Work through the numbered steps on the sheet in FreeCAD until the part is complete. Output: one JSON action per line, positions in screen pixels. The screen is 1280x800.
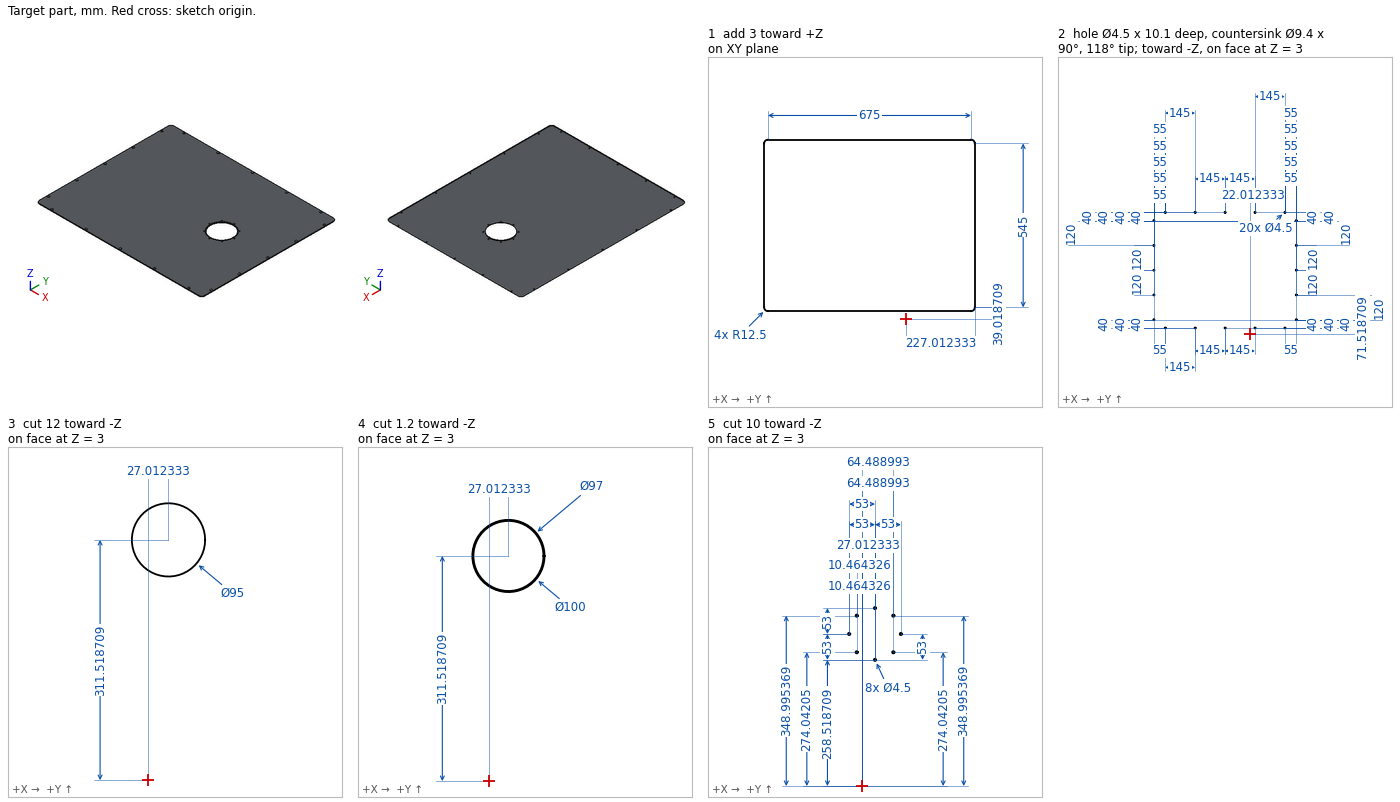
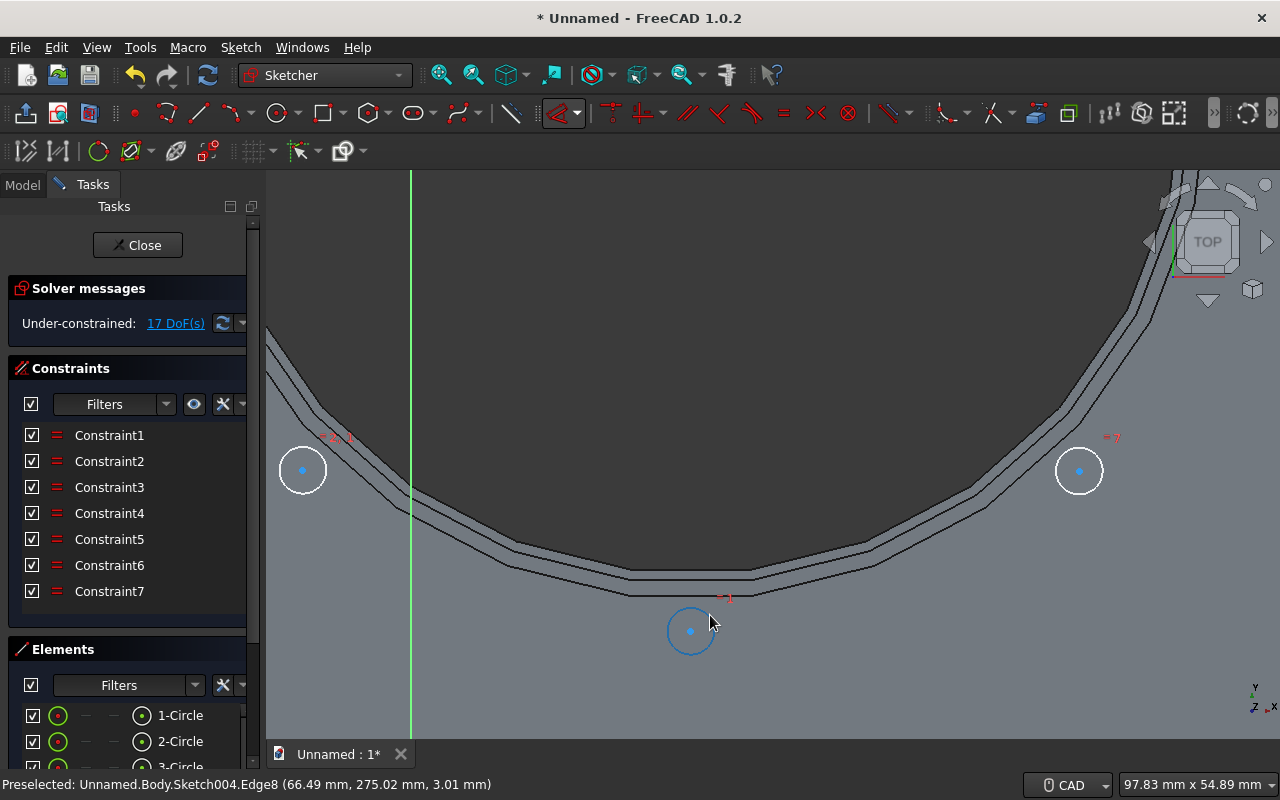
{"action": "left_click", "coordinate": [707, 615]}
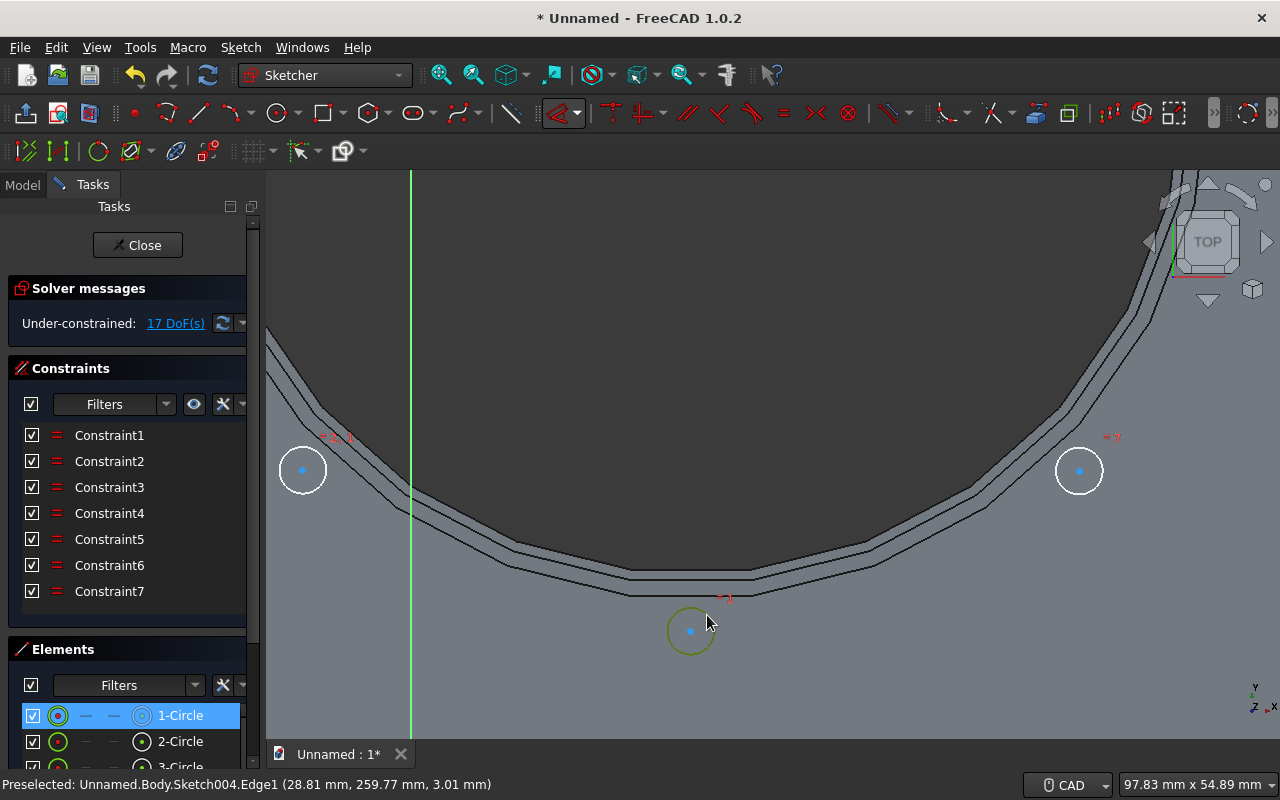
{"action": "left_click", "coordinate": [580, 114]}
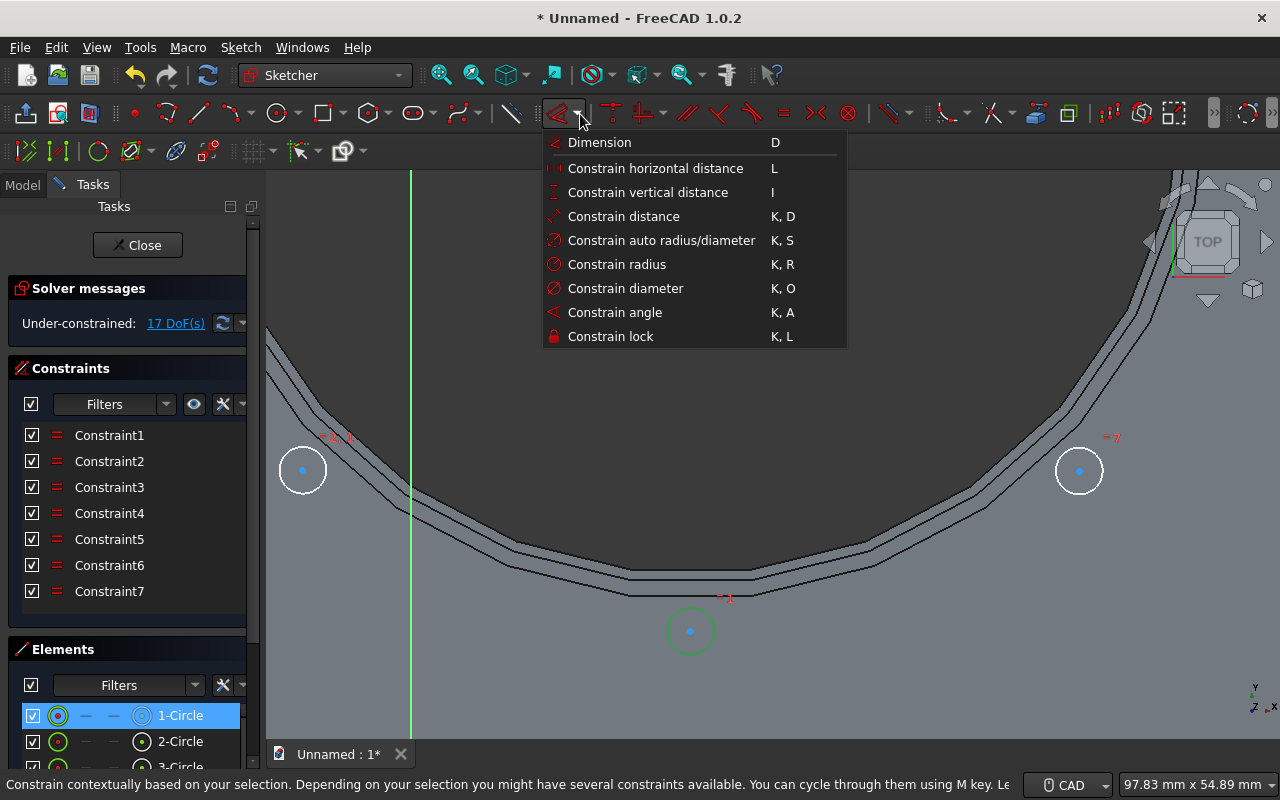
{"action": "left_click", "coordinate": [695, 288]}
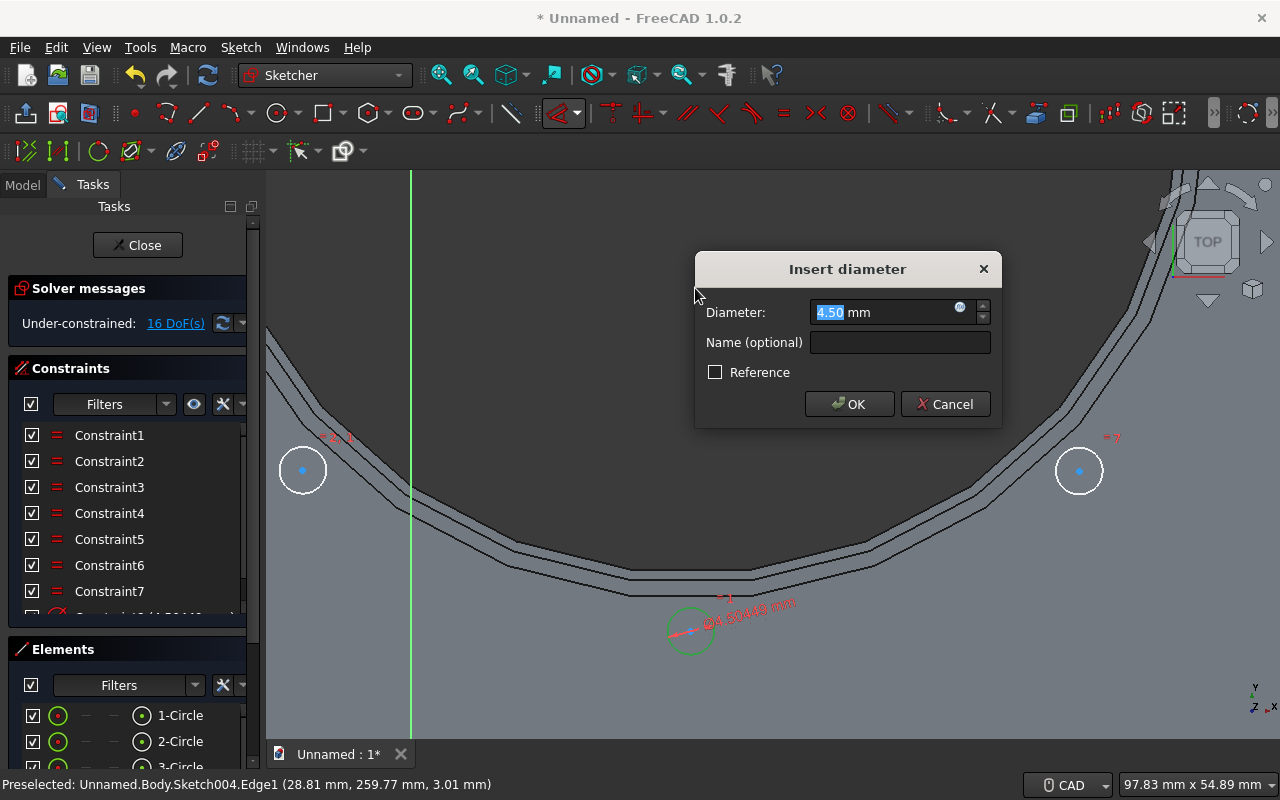
{"action": "type", "text": "4.5"}
{"action": "key", "text": "Return"}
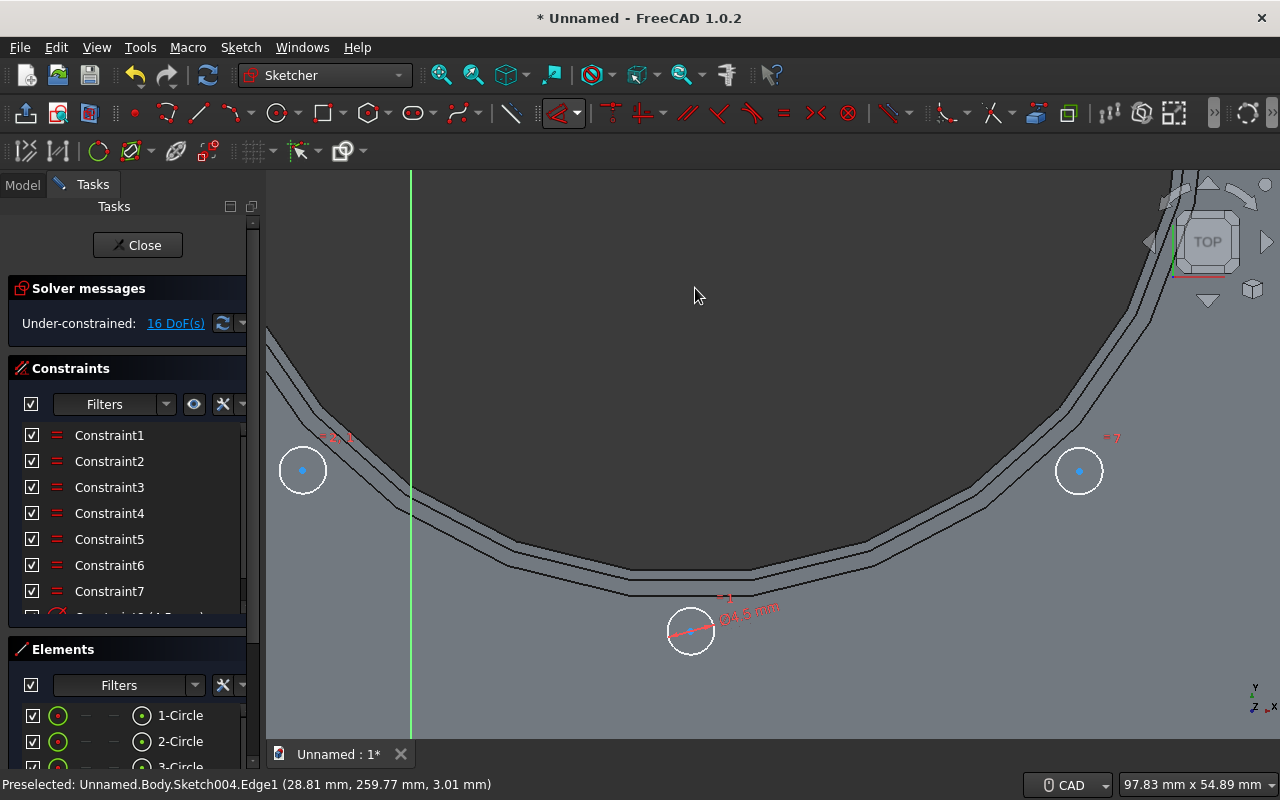
{"action": "left_click", "coordinate": [691, 631]}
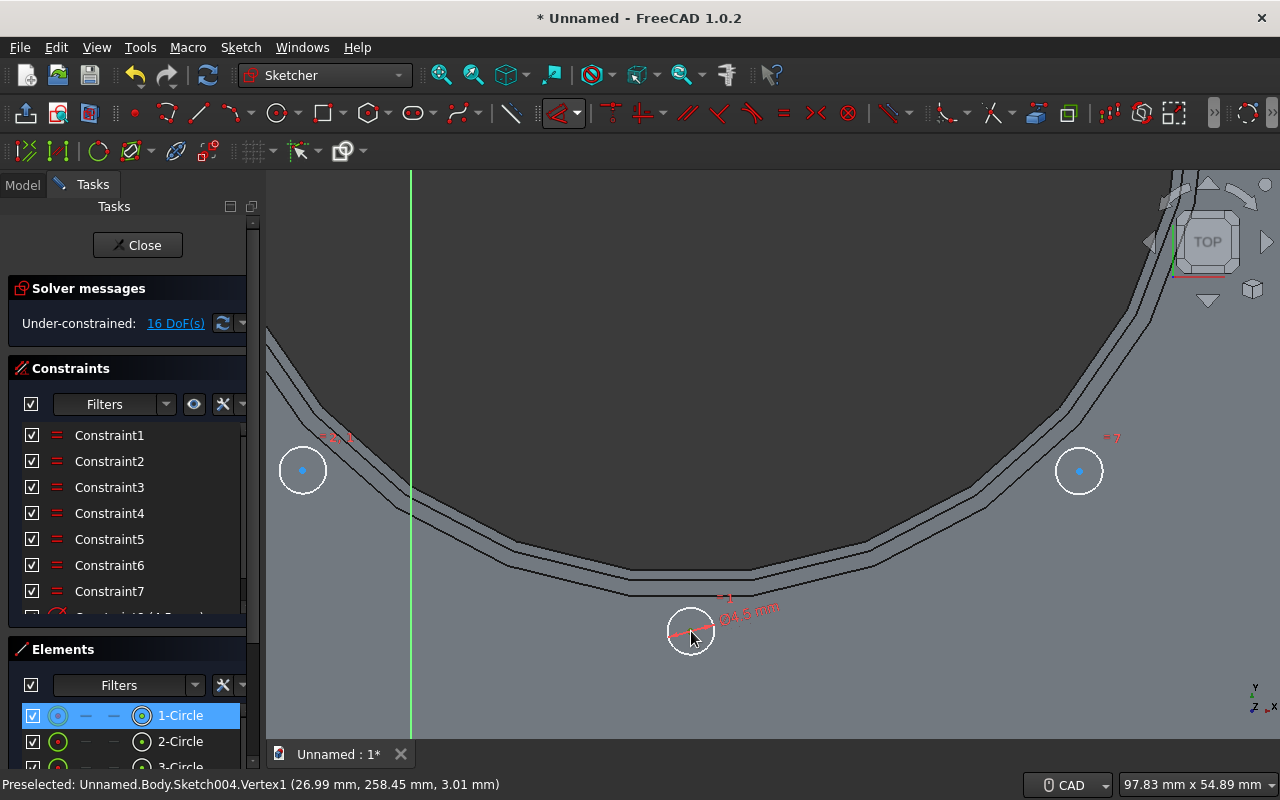
{"action": "scroll", "coordinate": [710, 615], "scroll_direction": "down", "scroll_amount": 6}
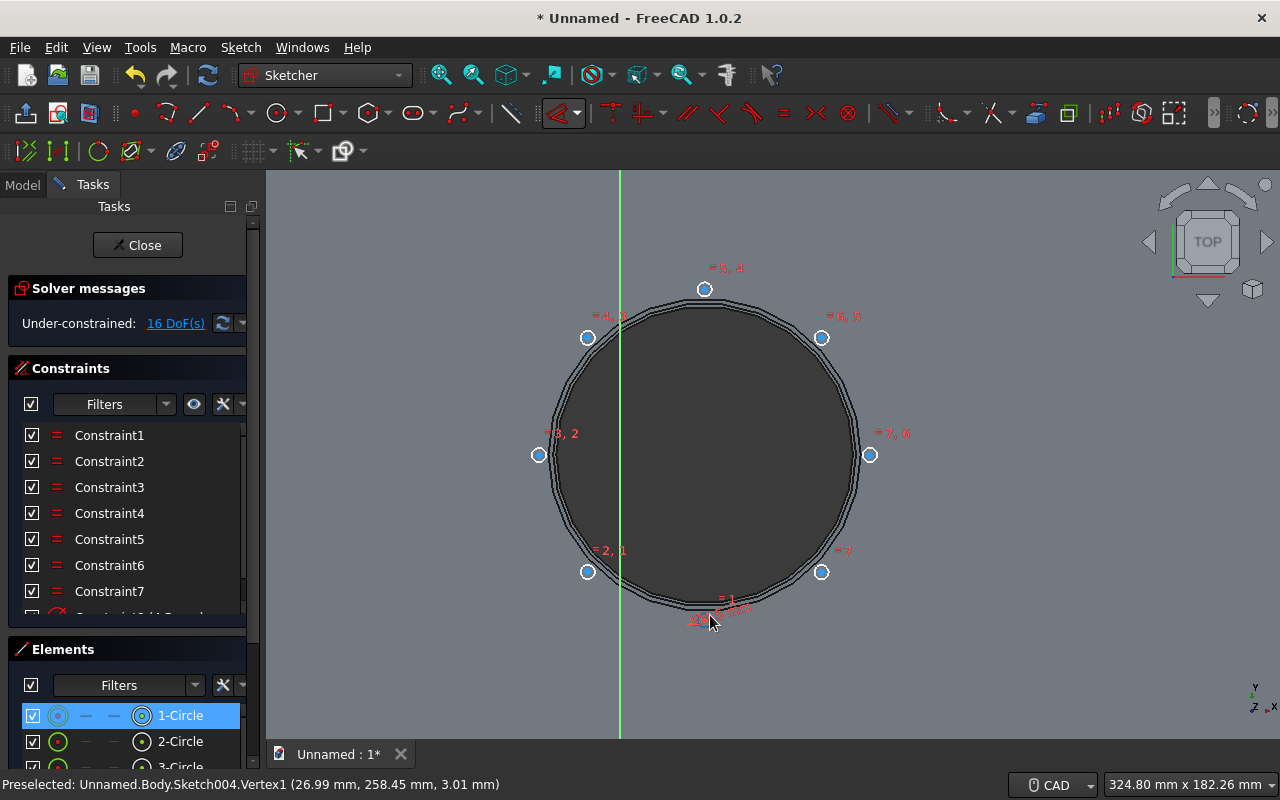
{"action": "left_click", "coordinate": [539, 455]}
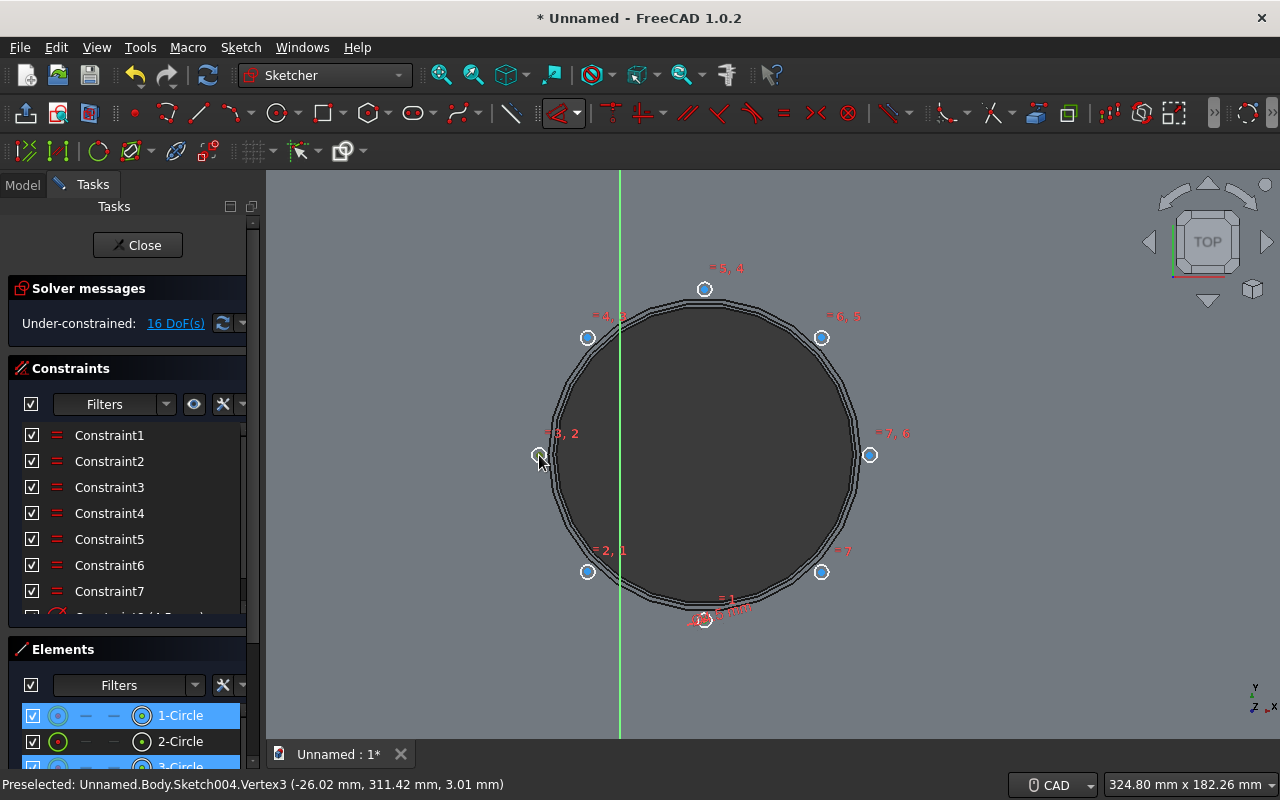
{"action": "left_click", "coordinate": [580, 114]}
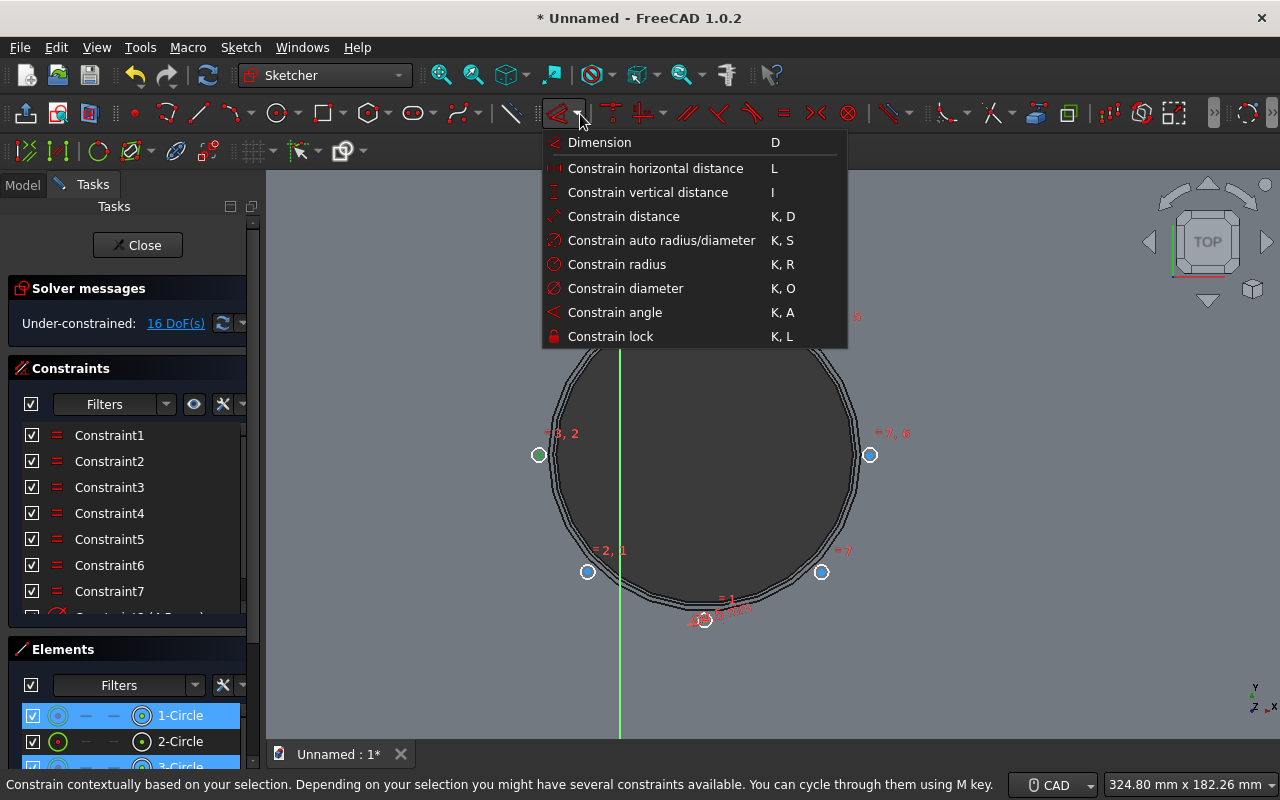
{"action": "left_click", "coordinate": [695, 168]}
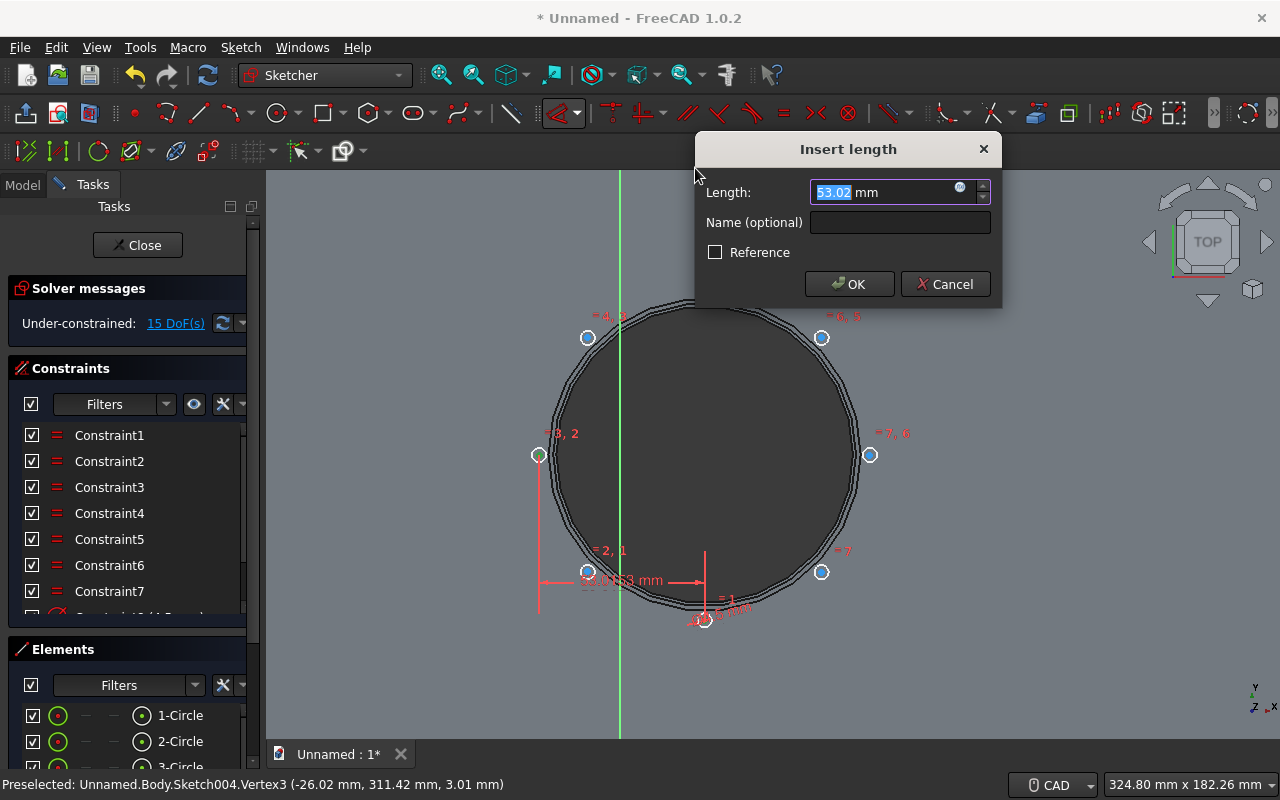
{"action": "type", "text": "53"}
{"action": "key", "text": "Return"}